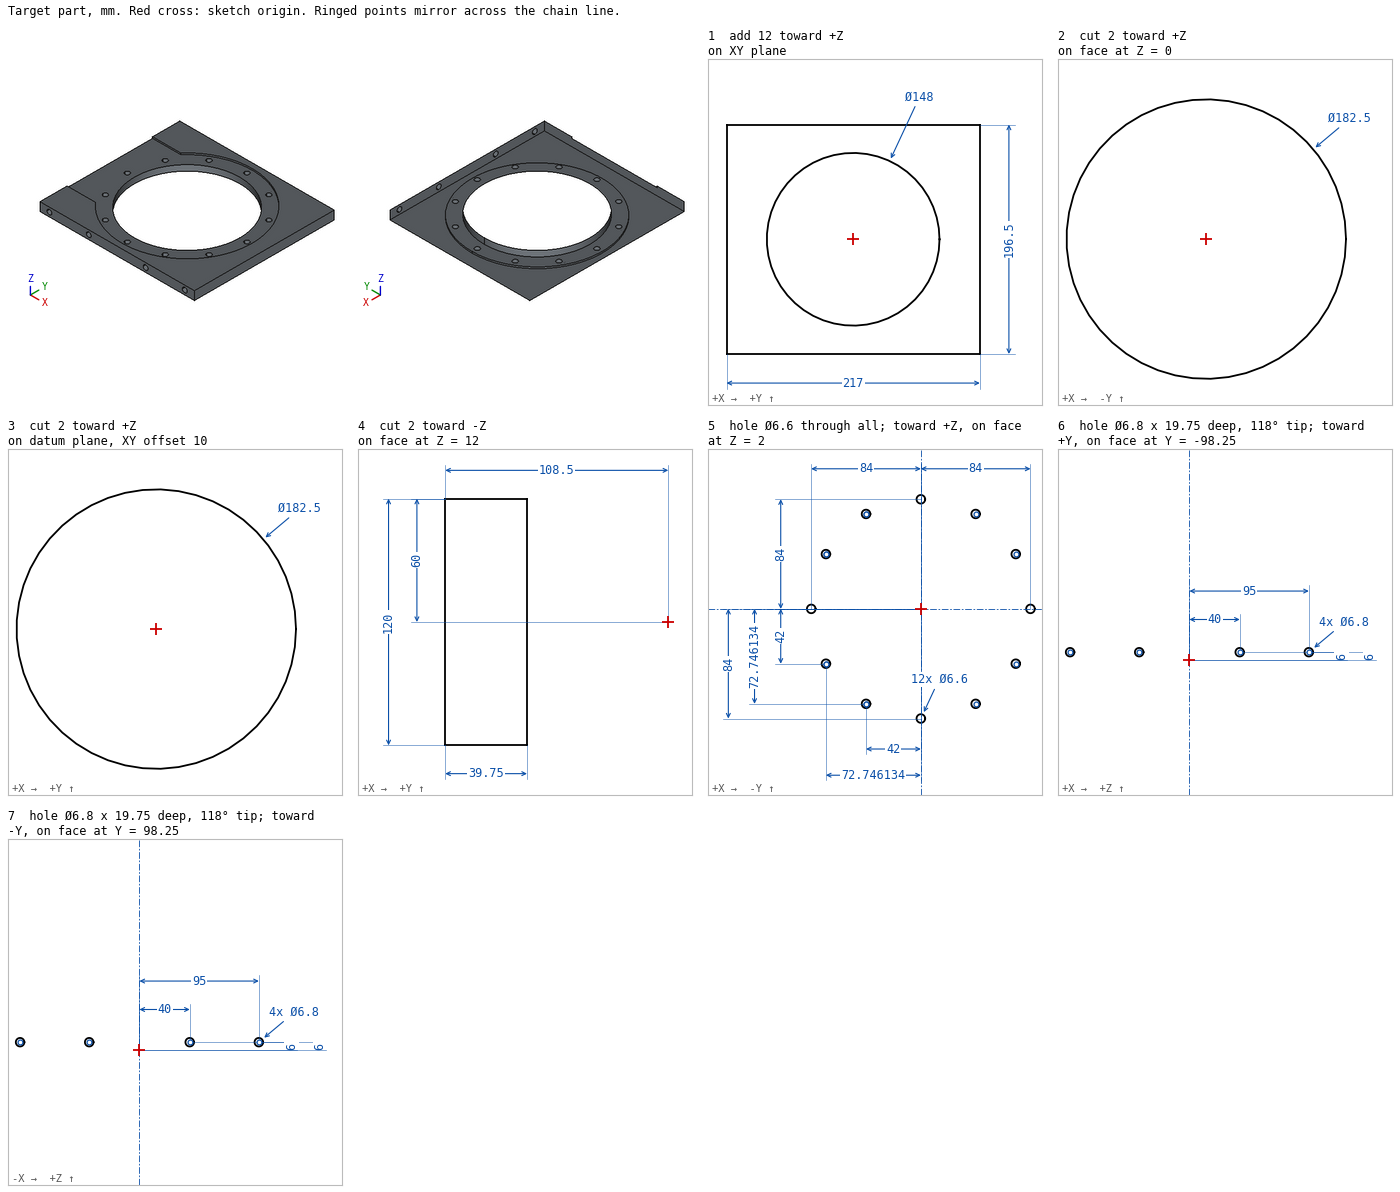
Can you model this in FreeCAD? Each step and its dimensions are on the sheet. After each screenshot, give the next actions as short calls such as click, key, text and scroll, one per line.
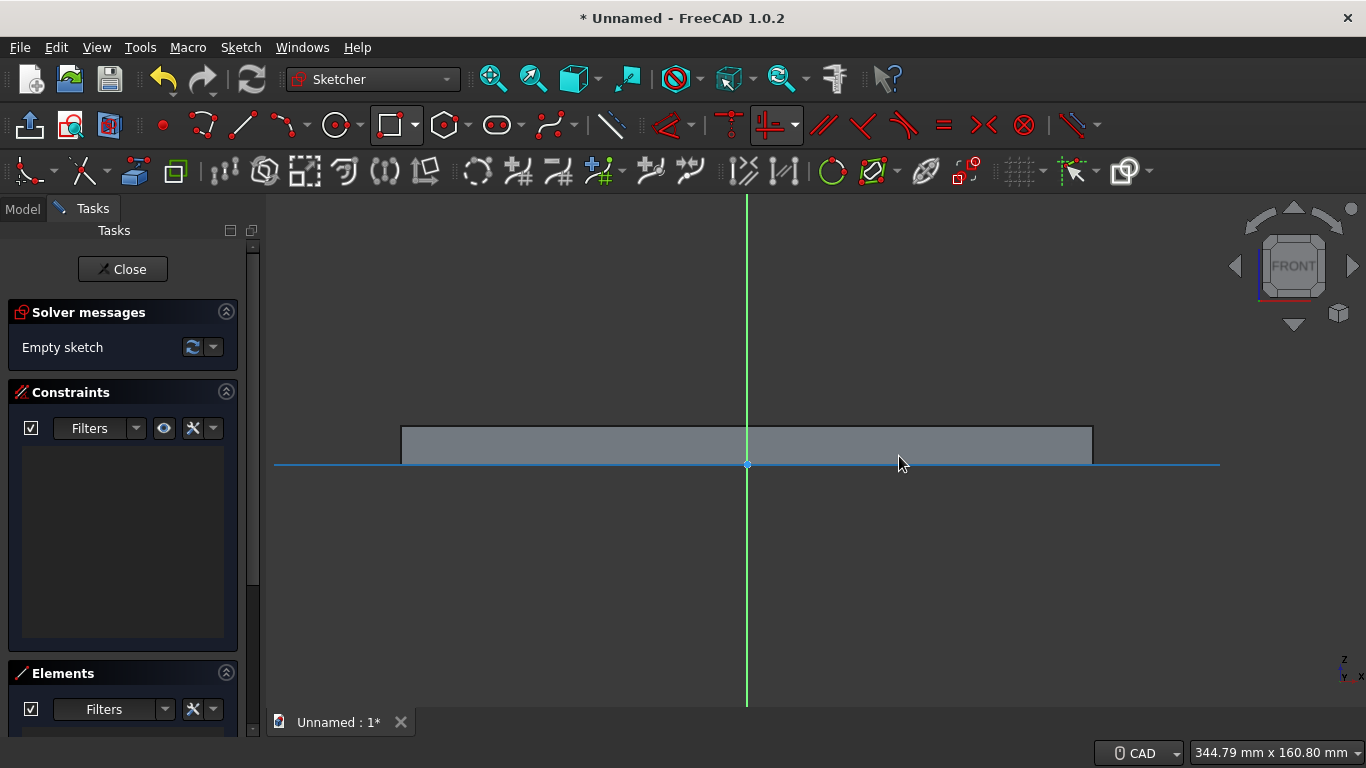
click(336, 126)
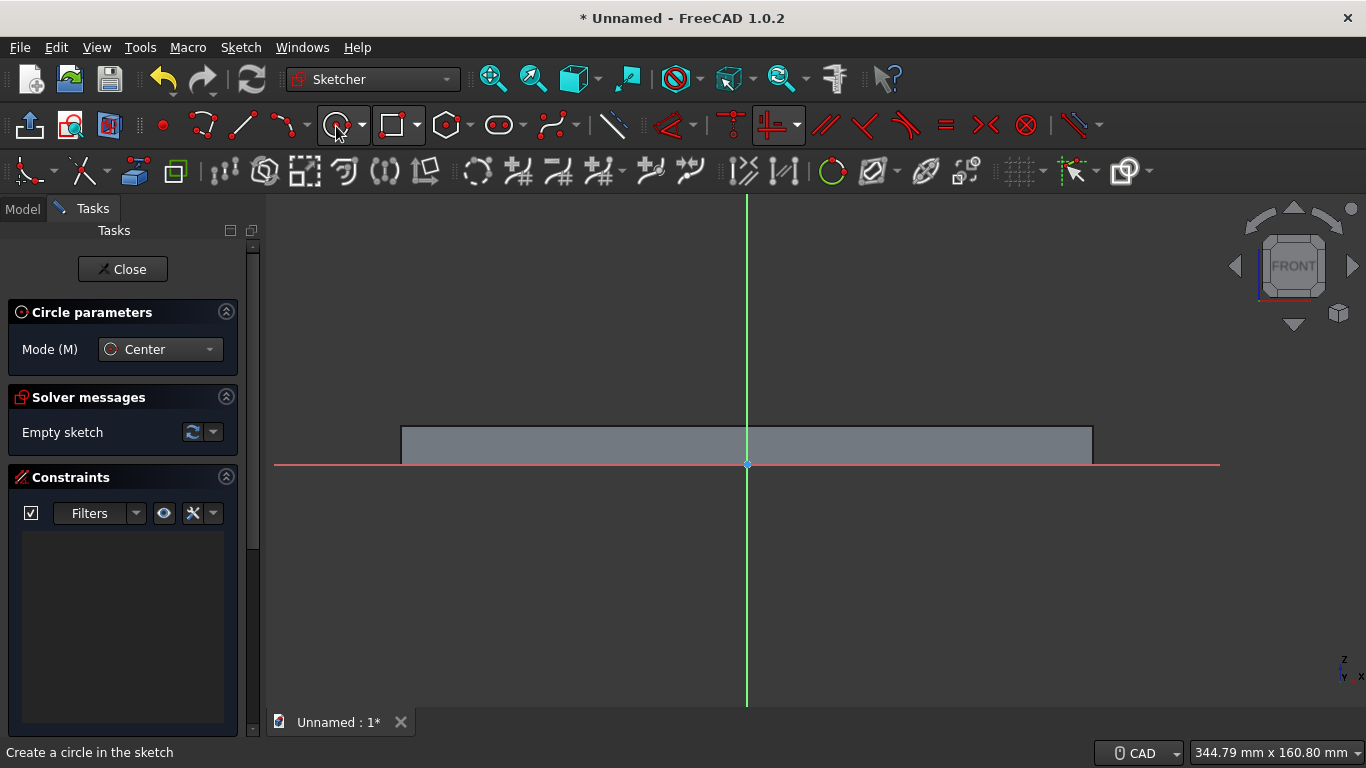
scroll(1050, 446, up, 4)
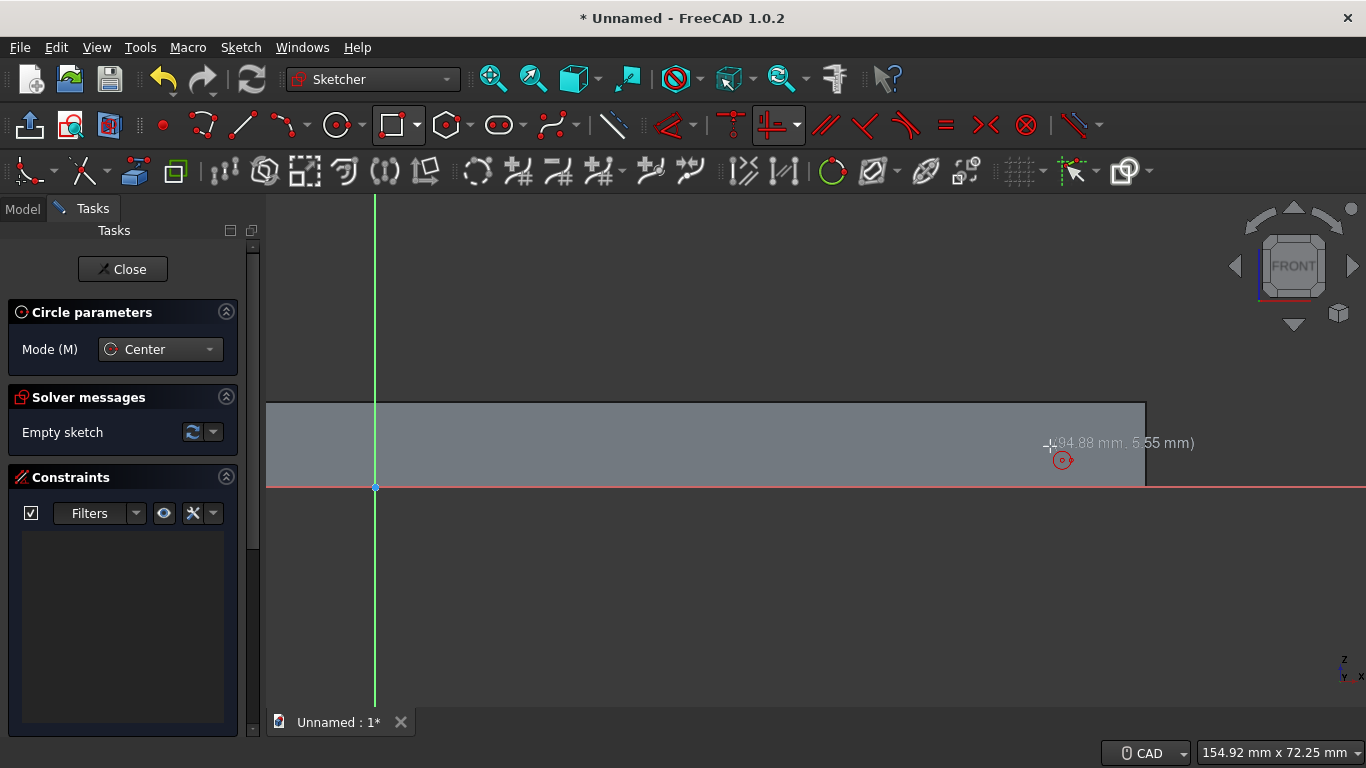
click(1050, 444)
click(1067, 427)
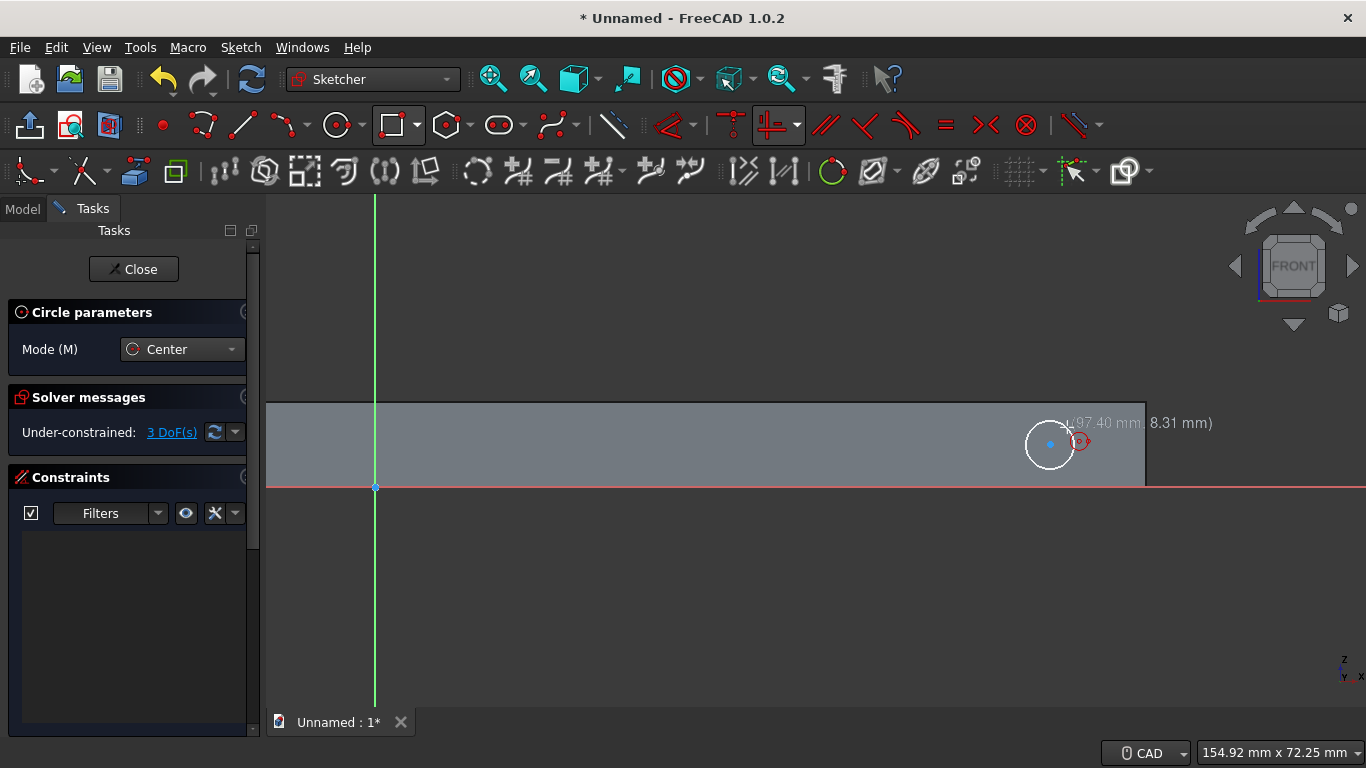
click(659, 444)
click(677, 427)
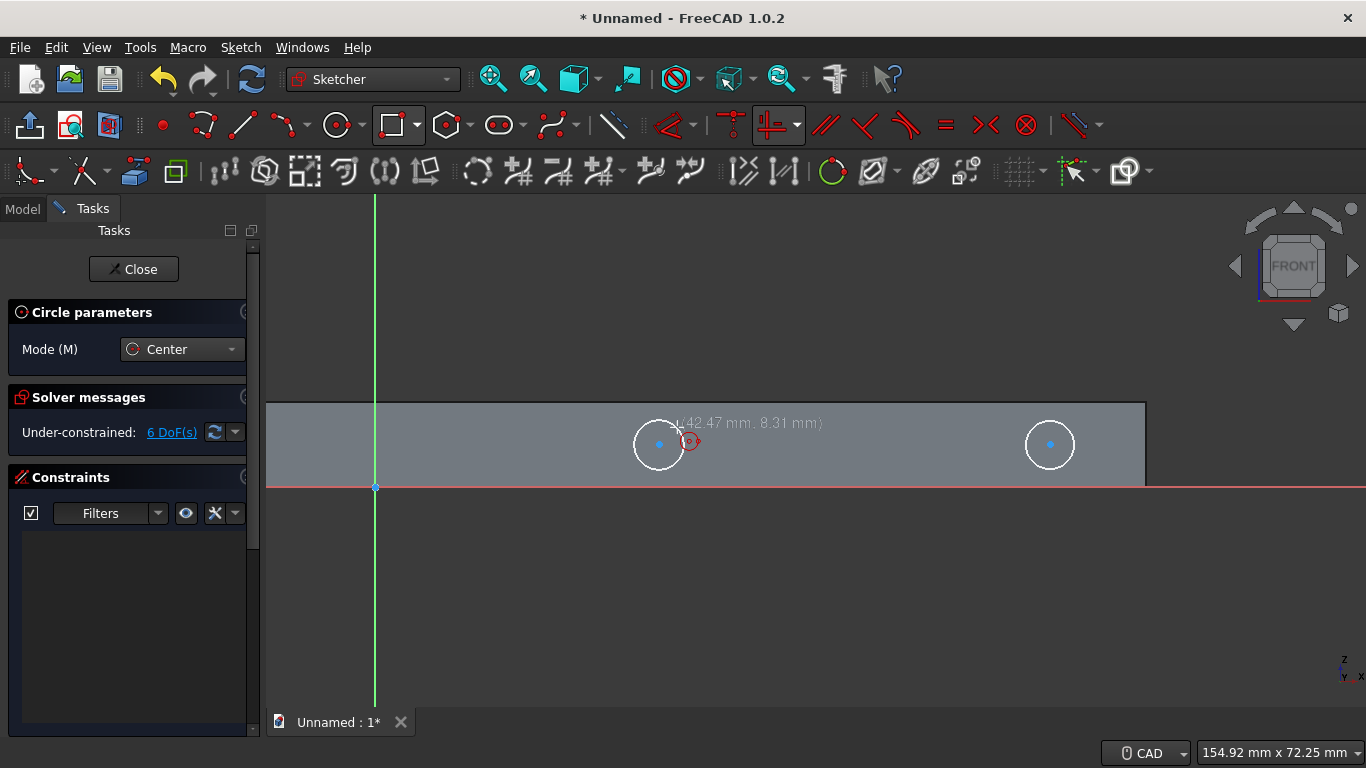
scroll(1051, 448, down, 4)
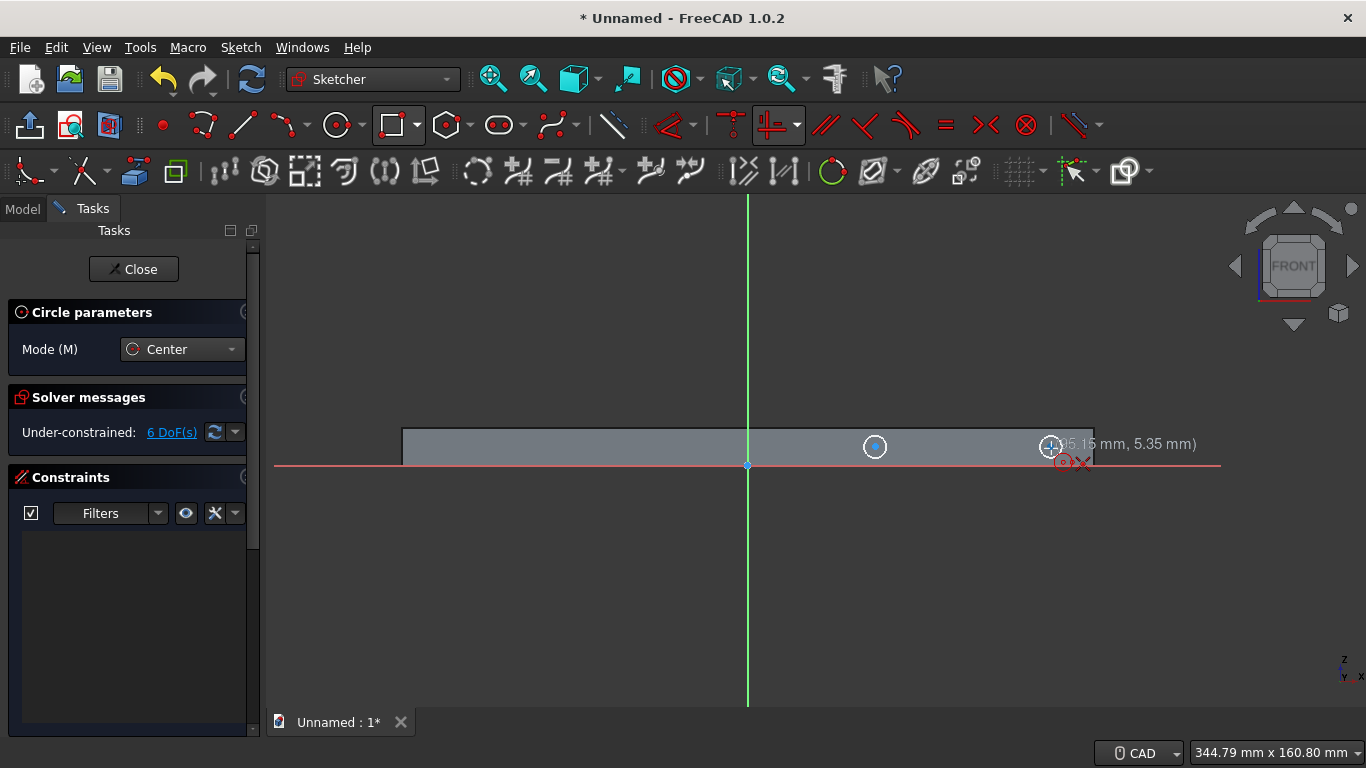
scroll(620, 447, up, 4)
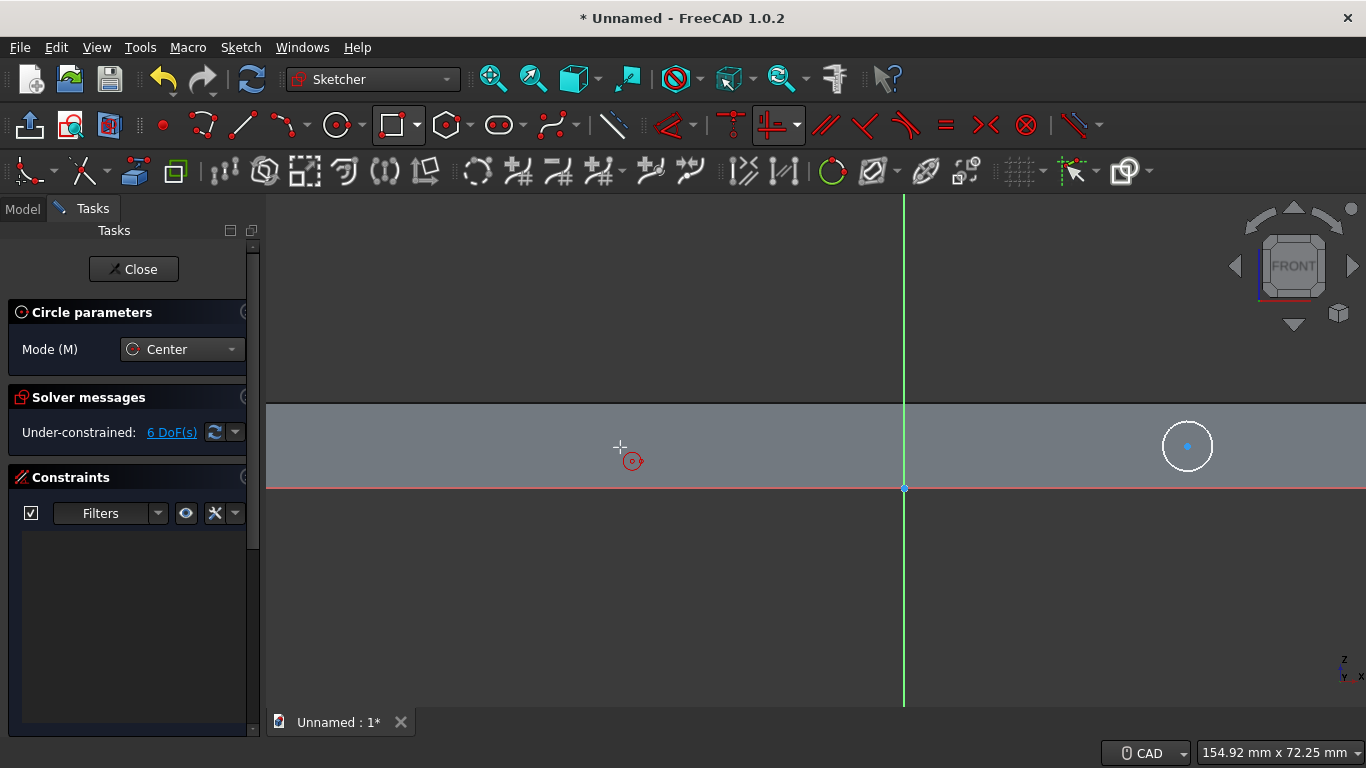
click(620, 446)
click(637, 429)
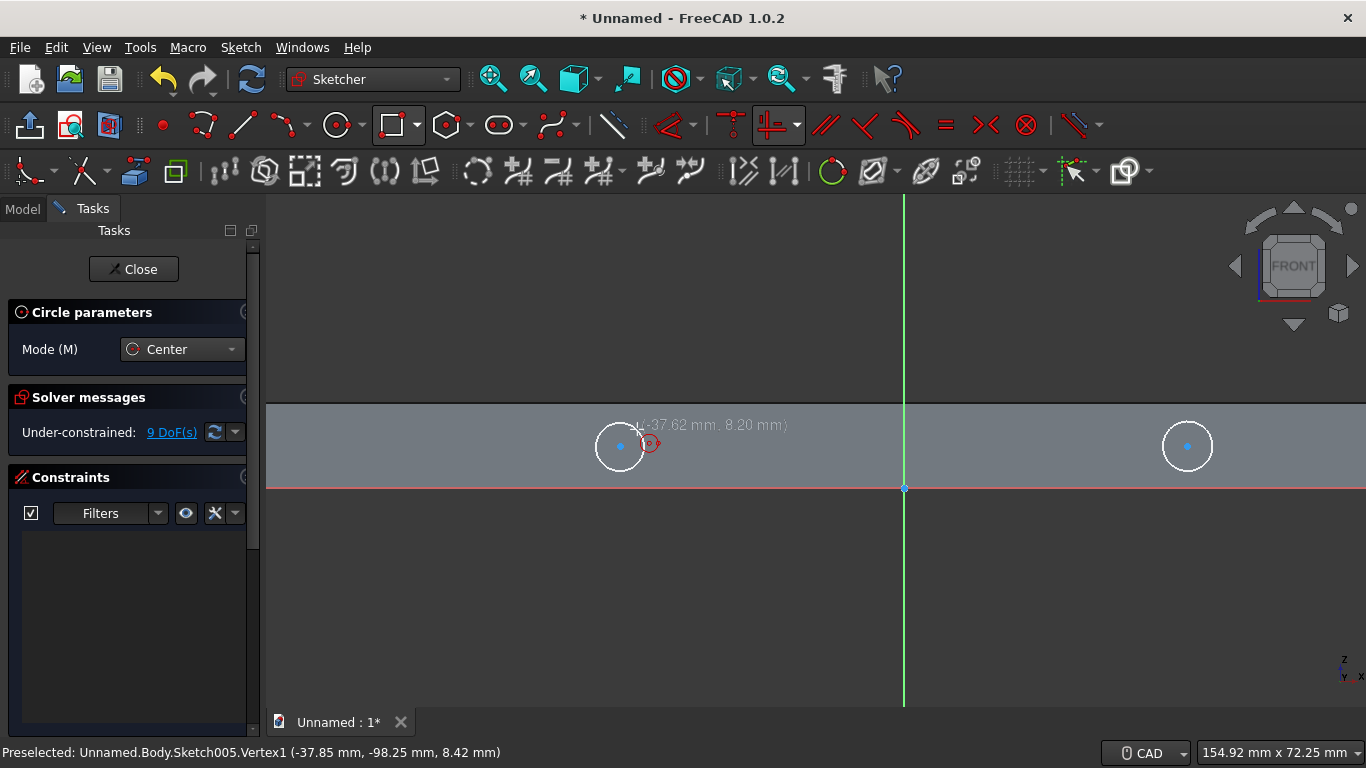
scroll(620, 447, down, 4)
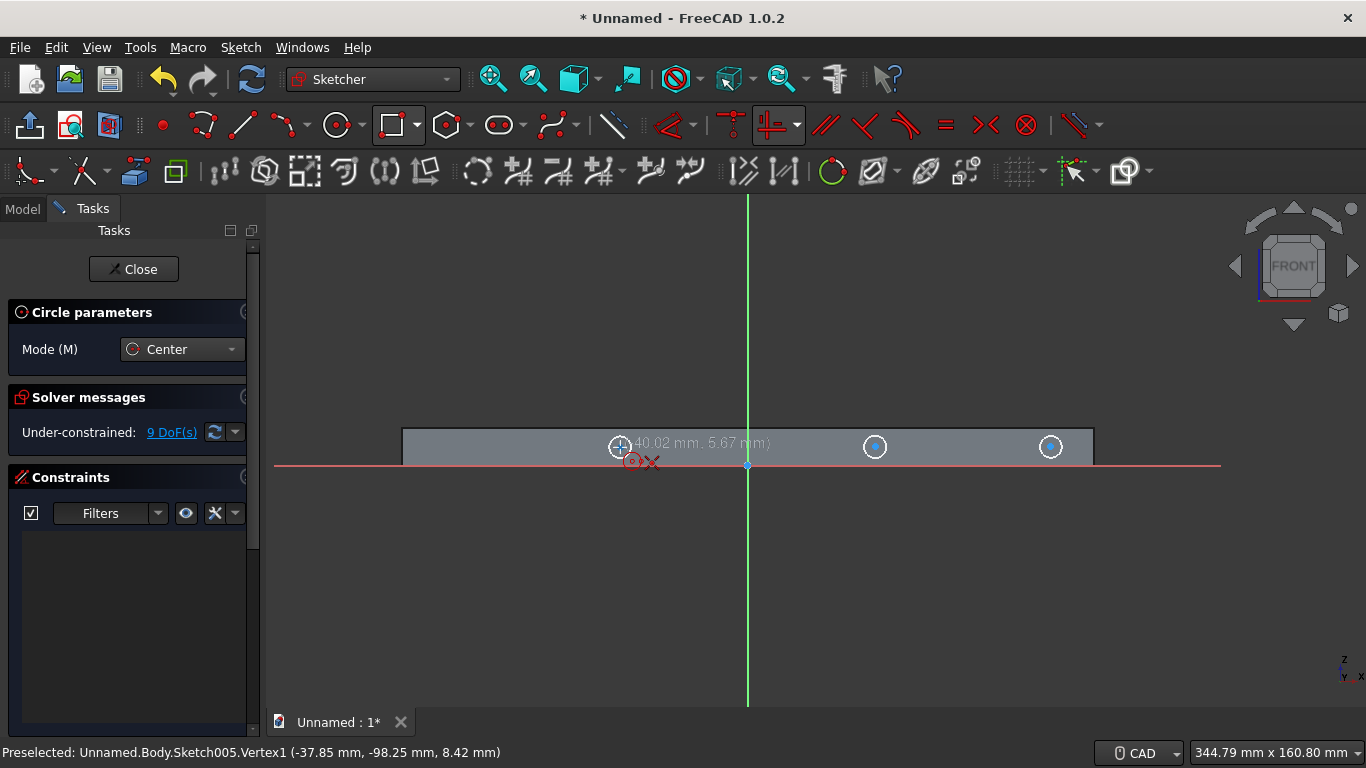
scroll(445, 447, up, 4)